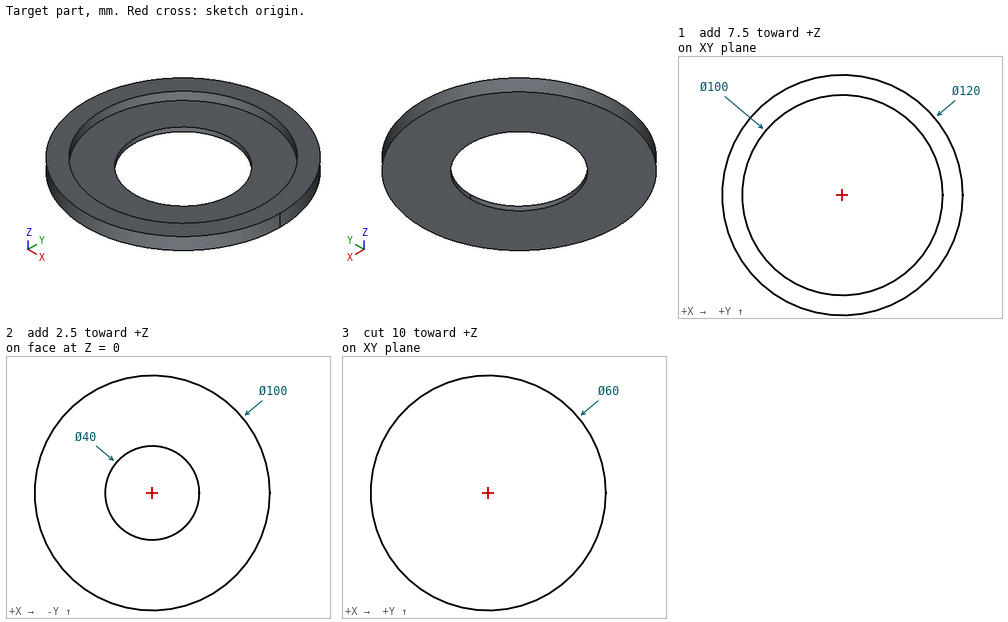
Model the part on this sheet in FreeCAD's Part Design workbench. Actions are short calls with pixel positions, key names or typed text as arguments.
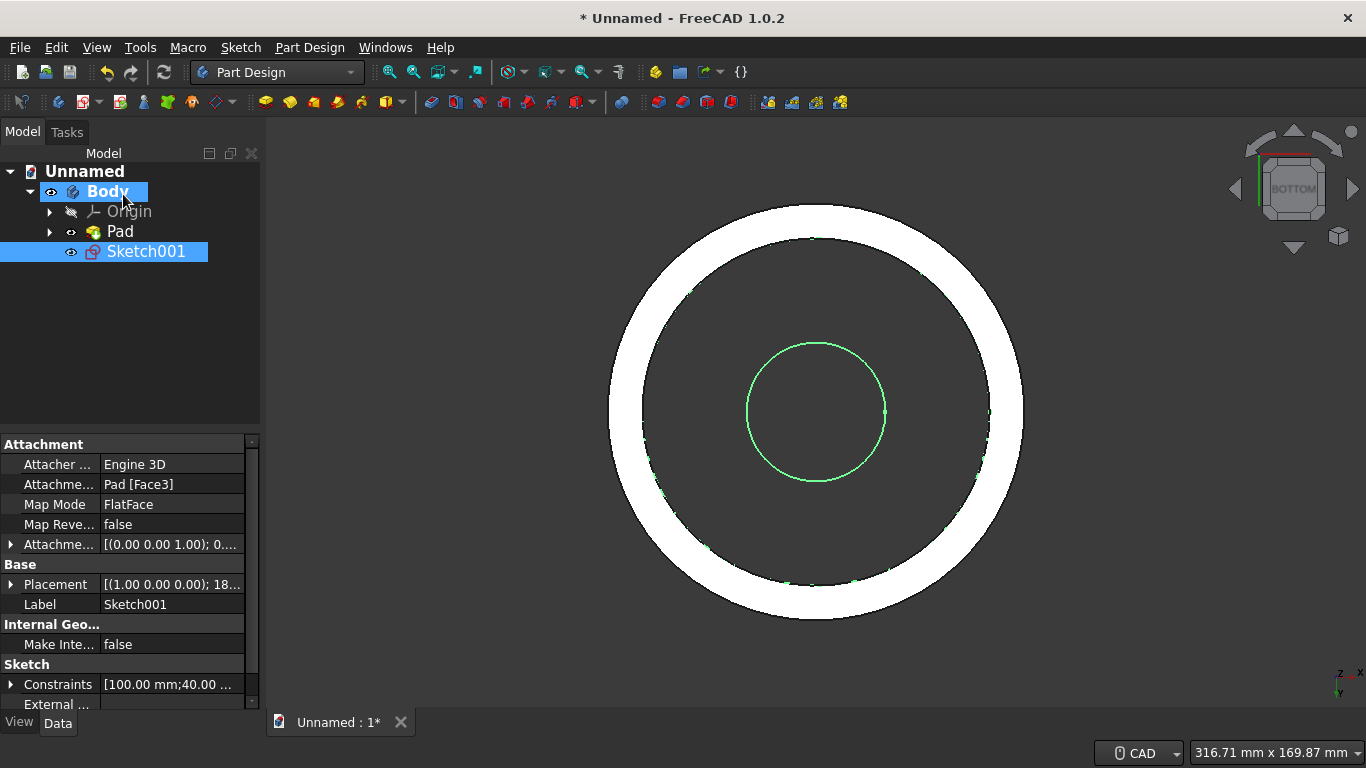
click(266, 102)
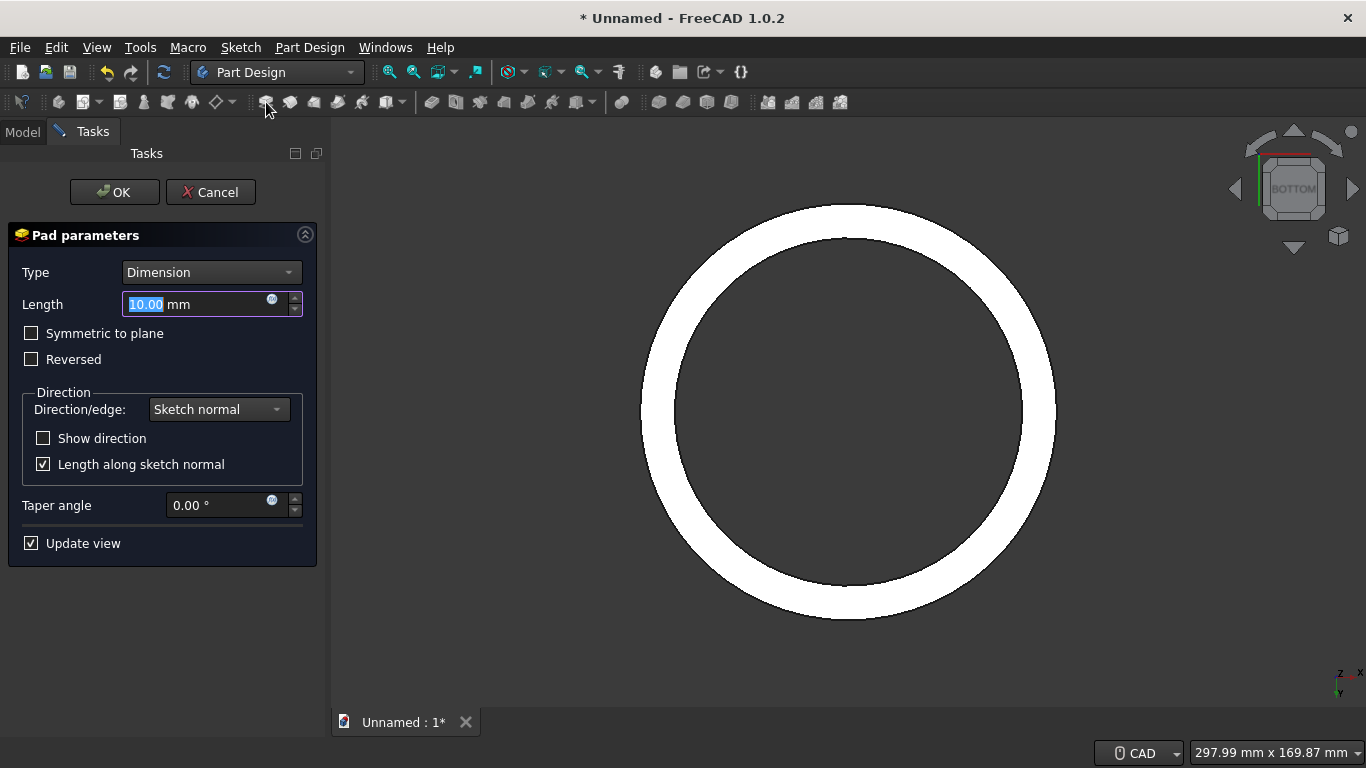
text(2.5)
key(Tab)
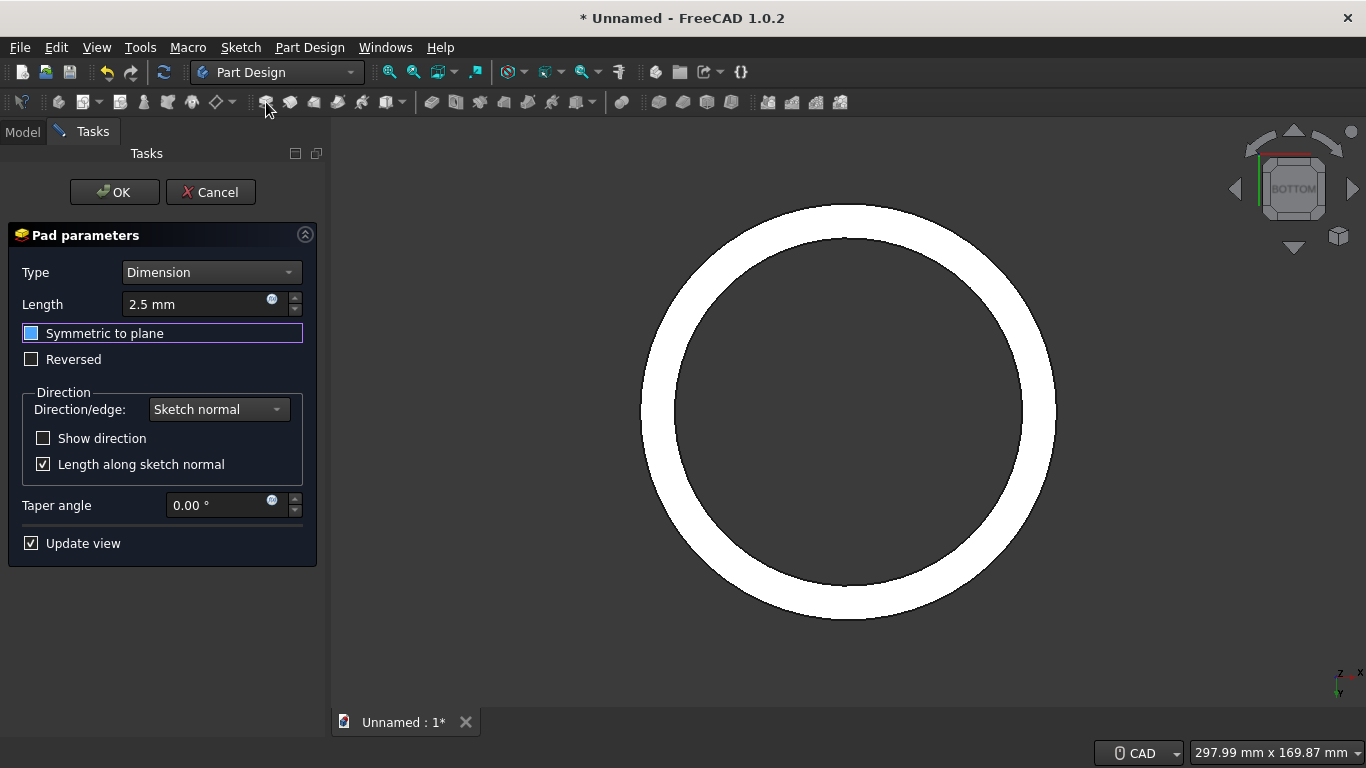
click(30, 359)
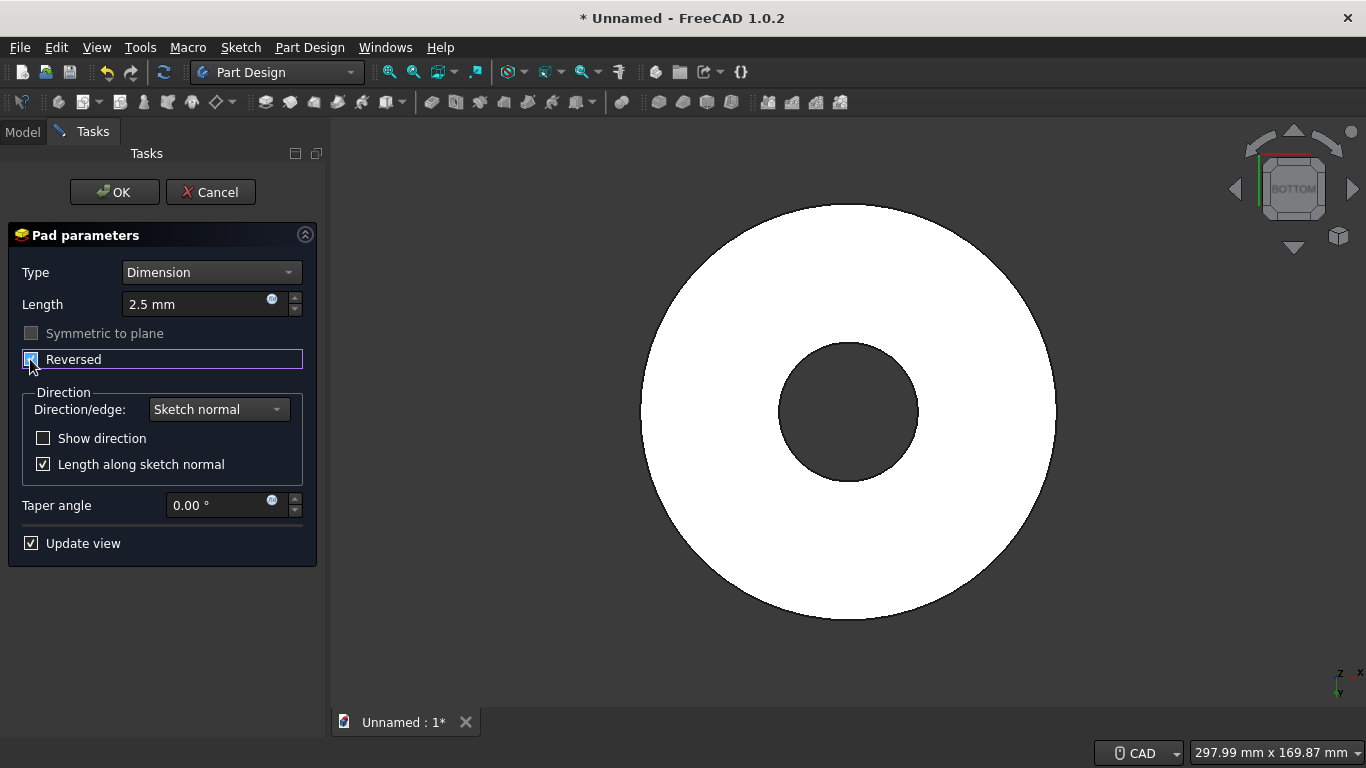
click(115, 192)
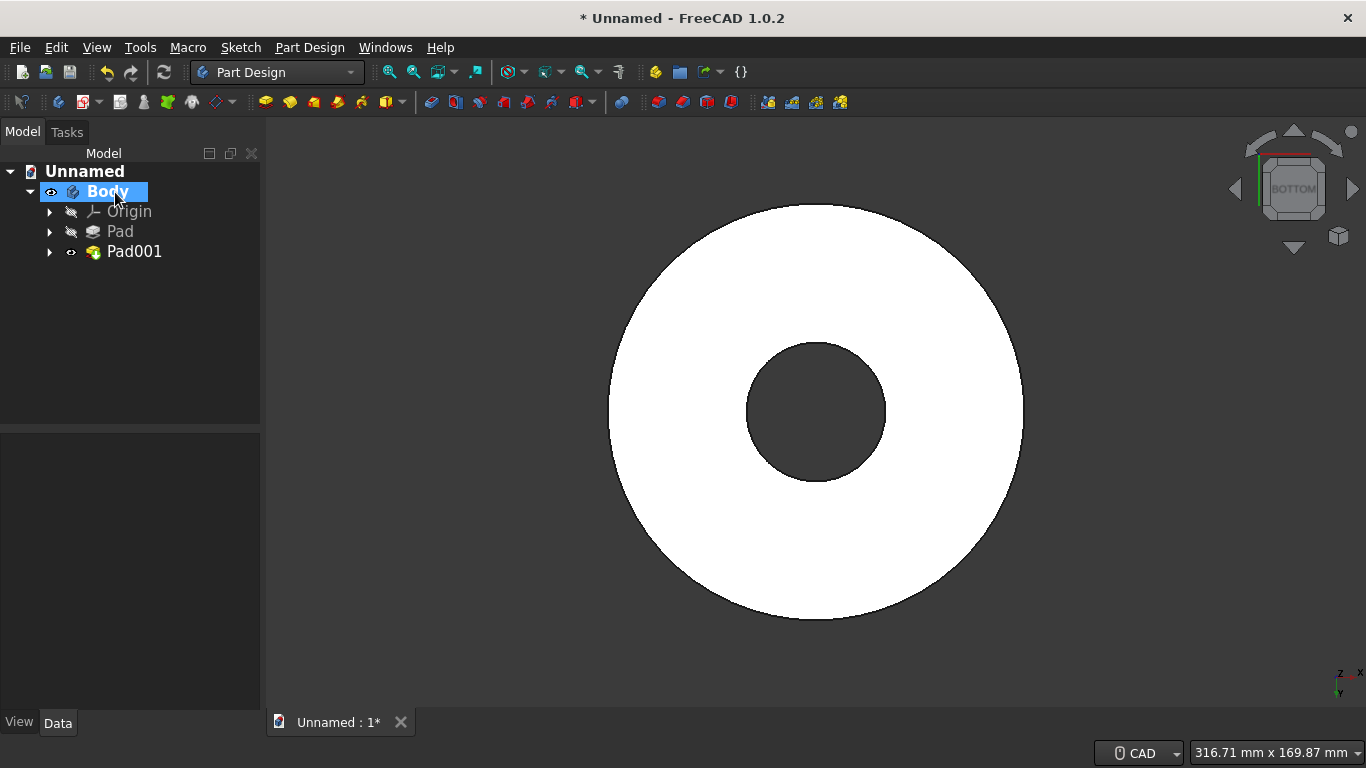
click(84, 102)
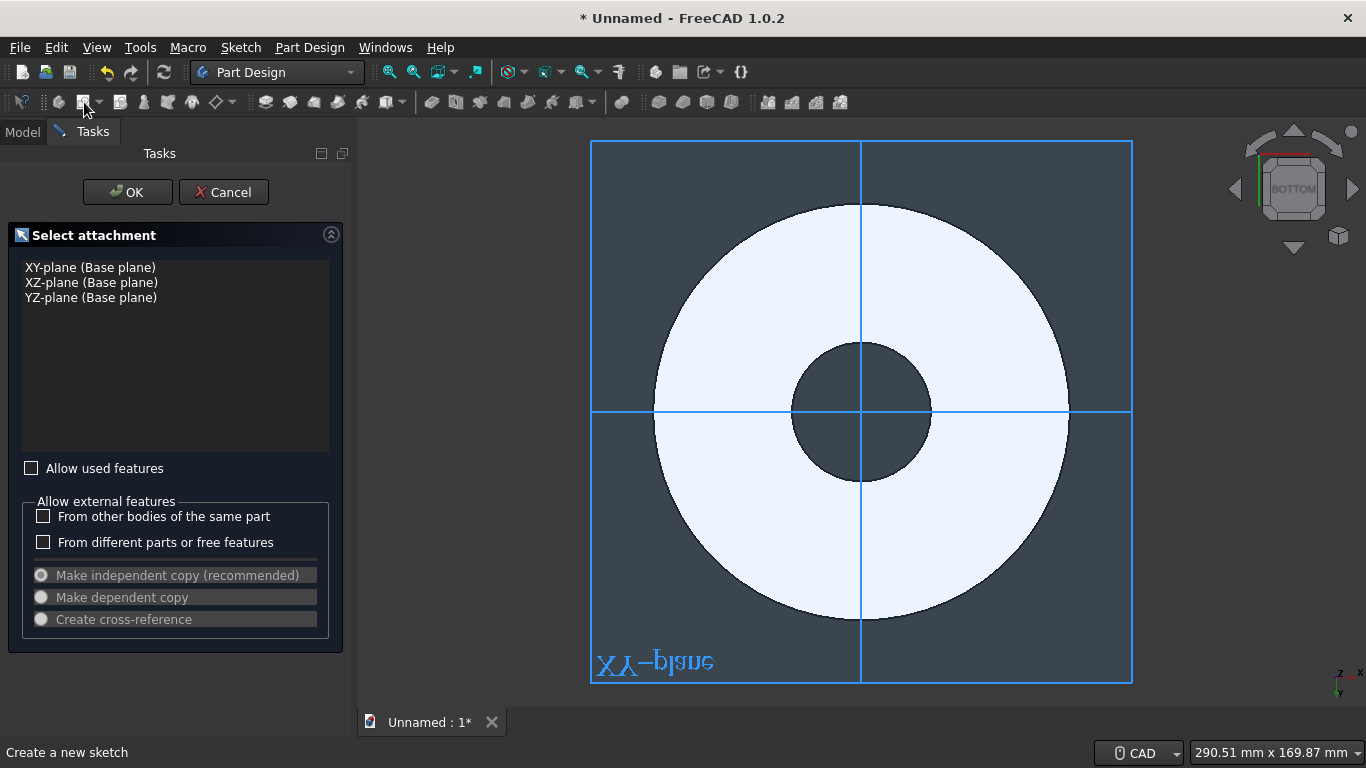
click(82, 268)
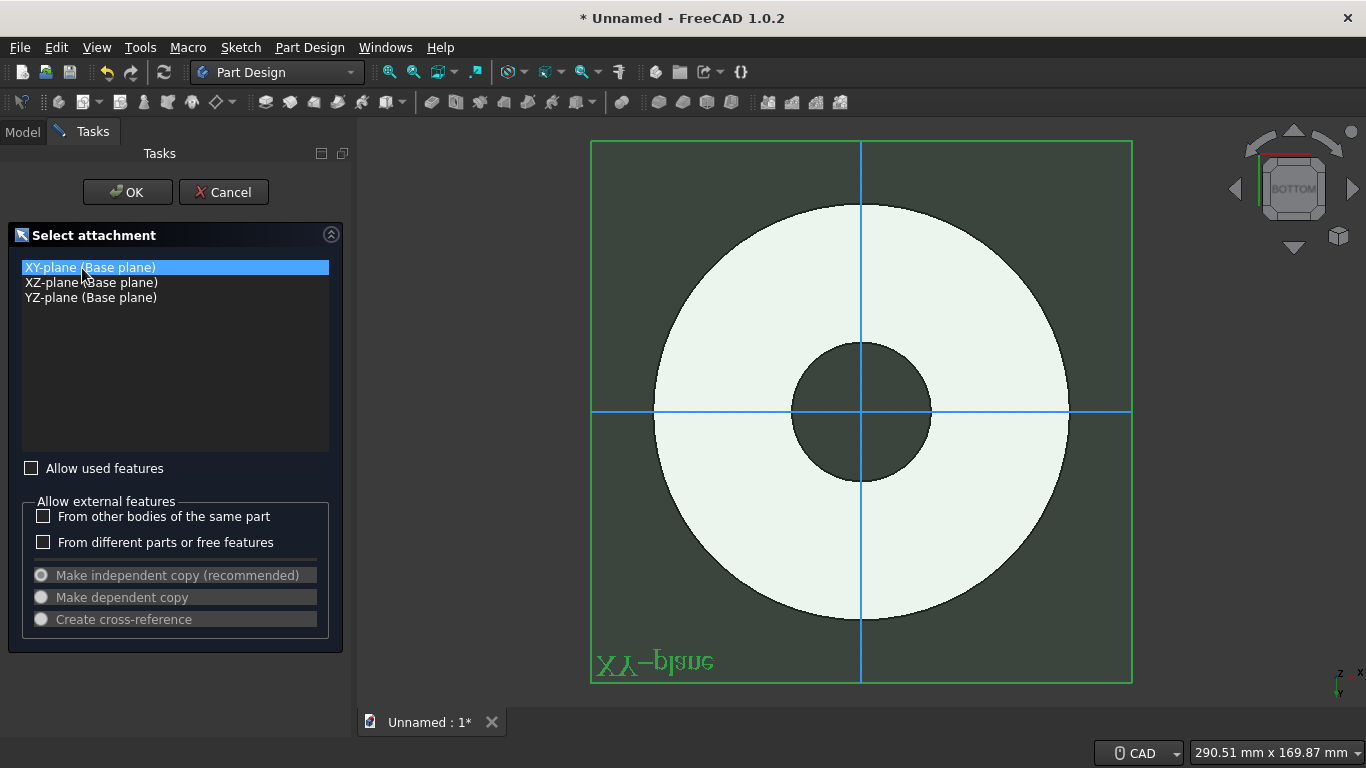
click(128, 192)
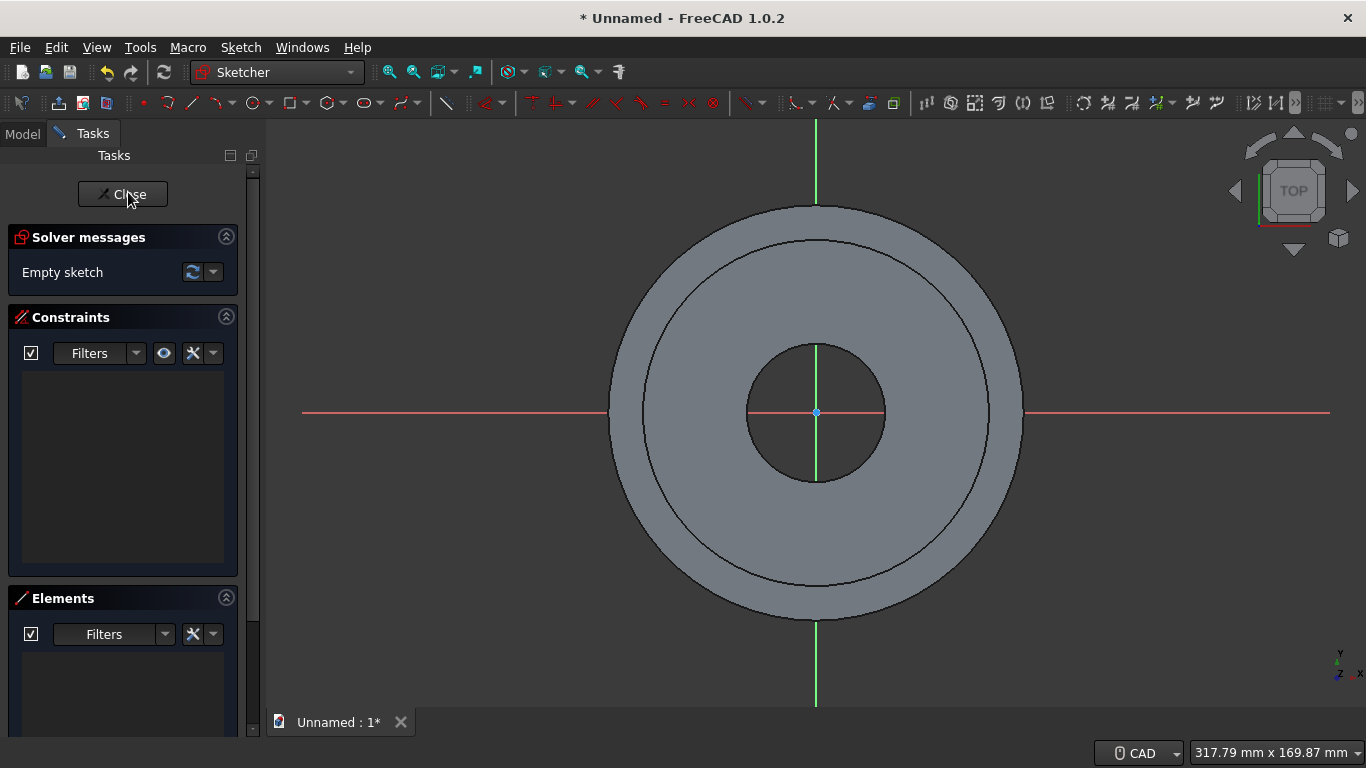
click(108, 104)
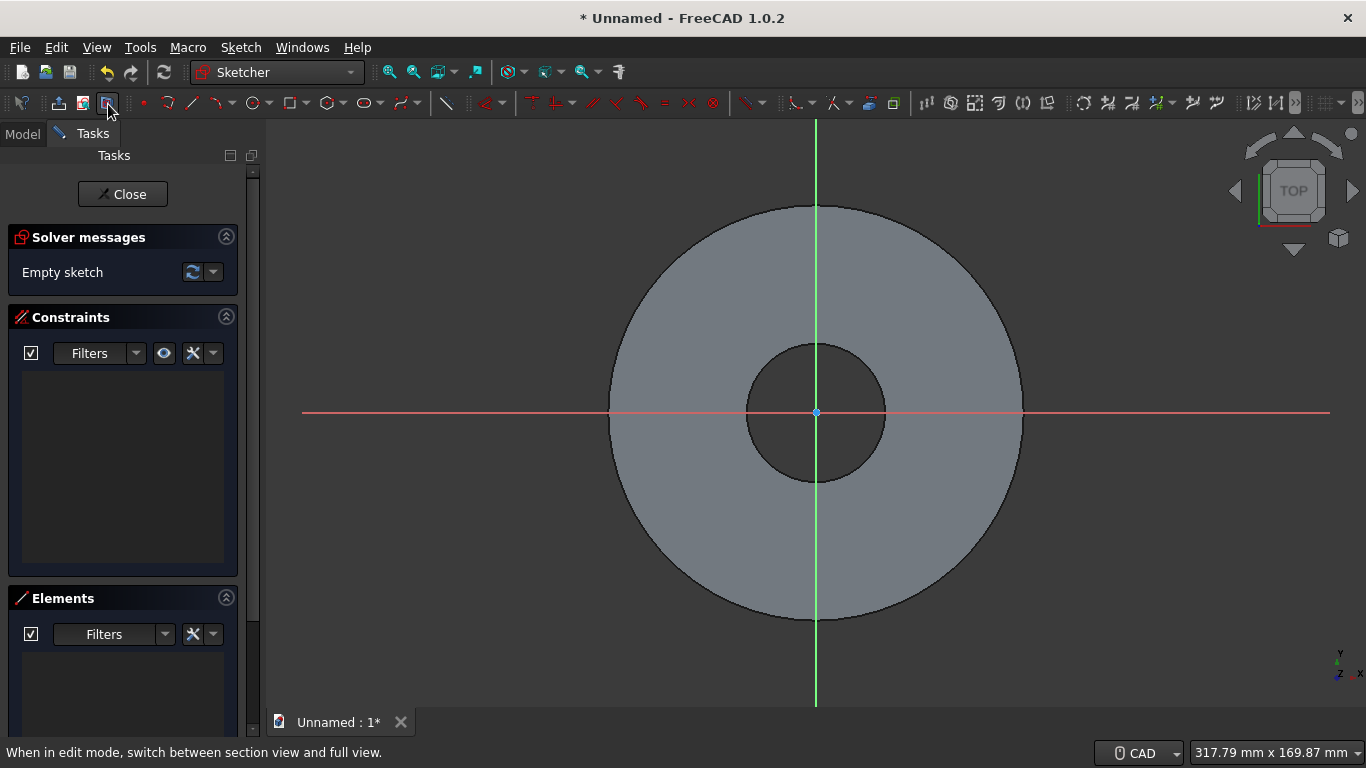
scroll(899, 413, up, 3)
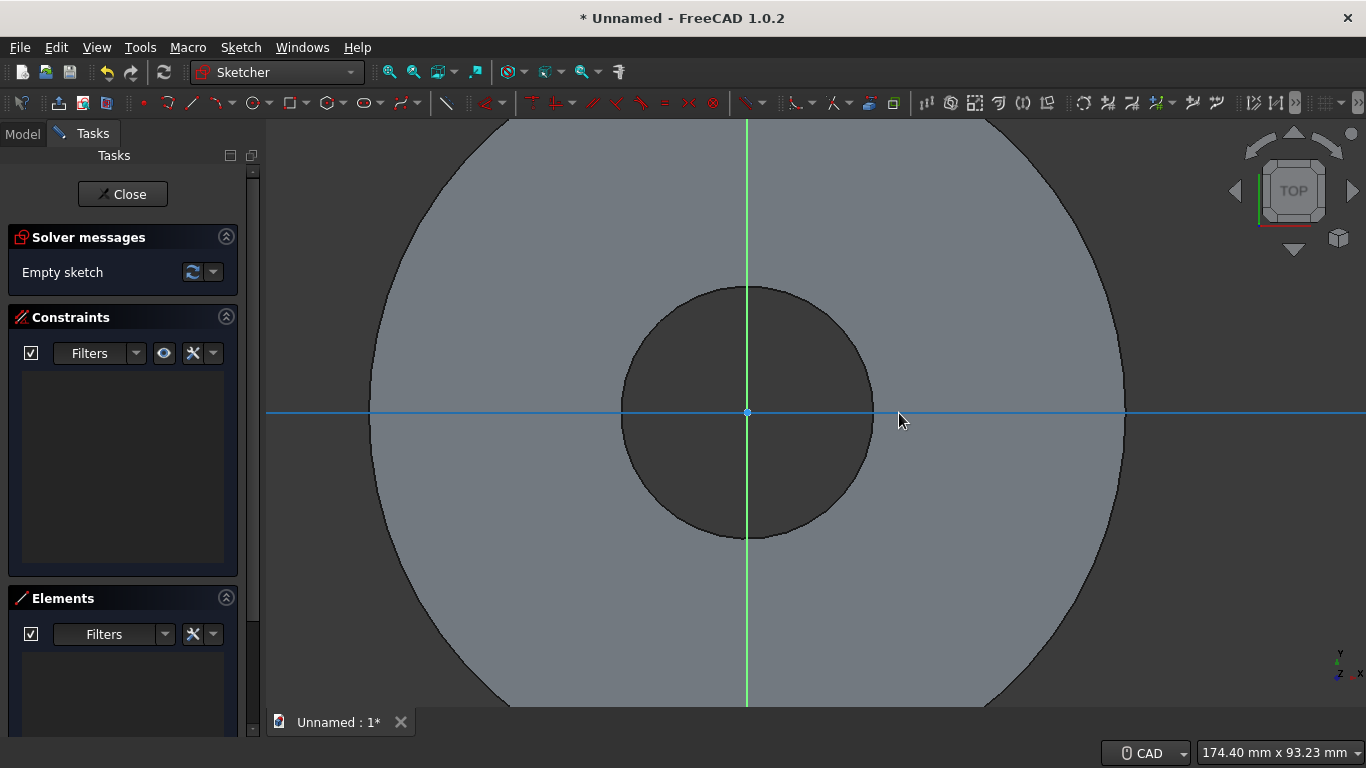
click(254, 104)